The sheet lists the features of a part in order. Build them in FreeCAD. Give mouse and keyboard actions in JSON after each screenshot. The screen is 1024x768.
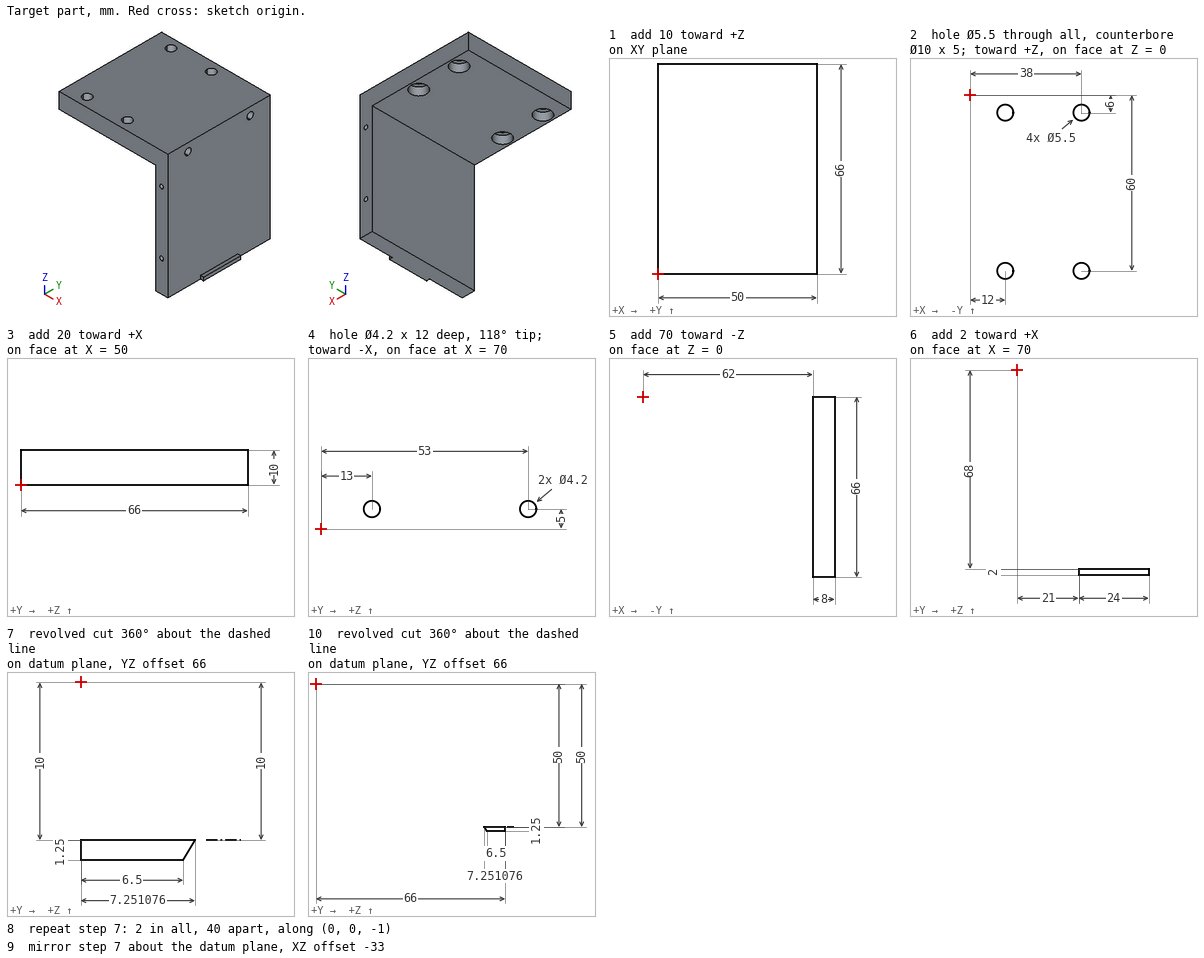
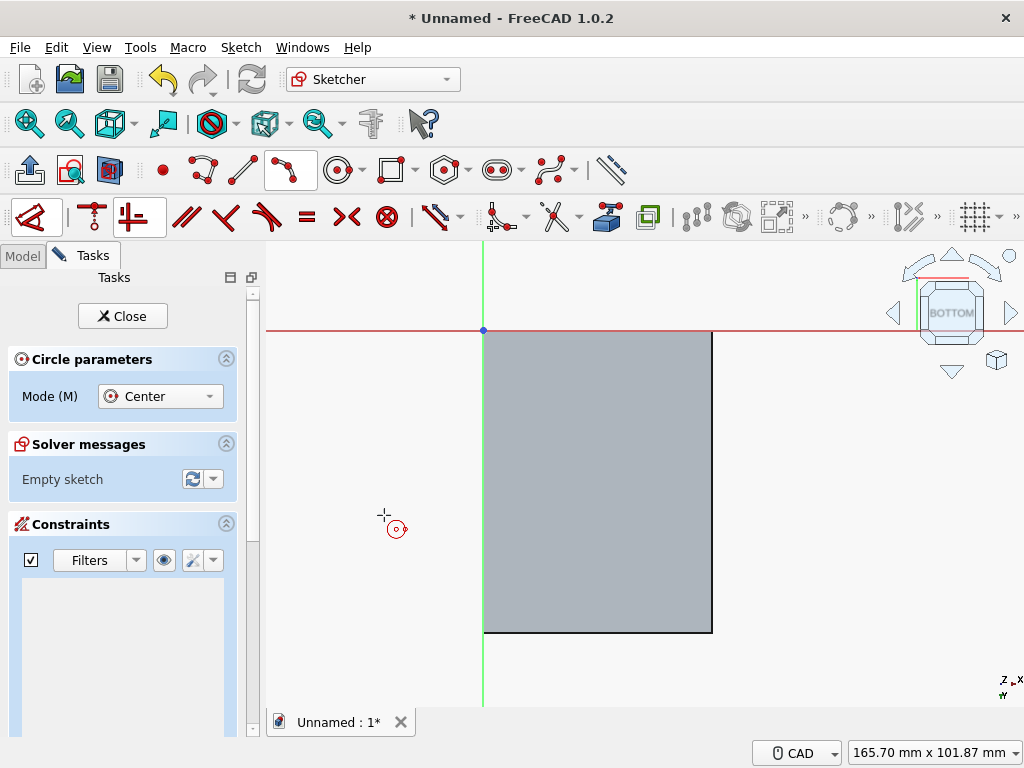
{"action": "scroll", "coordinate": [657, 358], "scroll_direction": "up", "scroll_amount": 3}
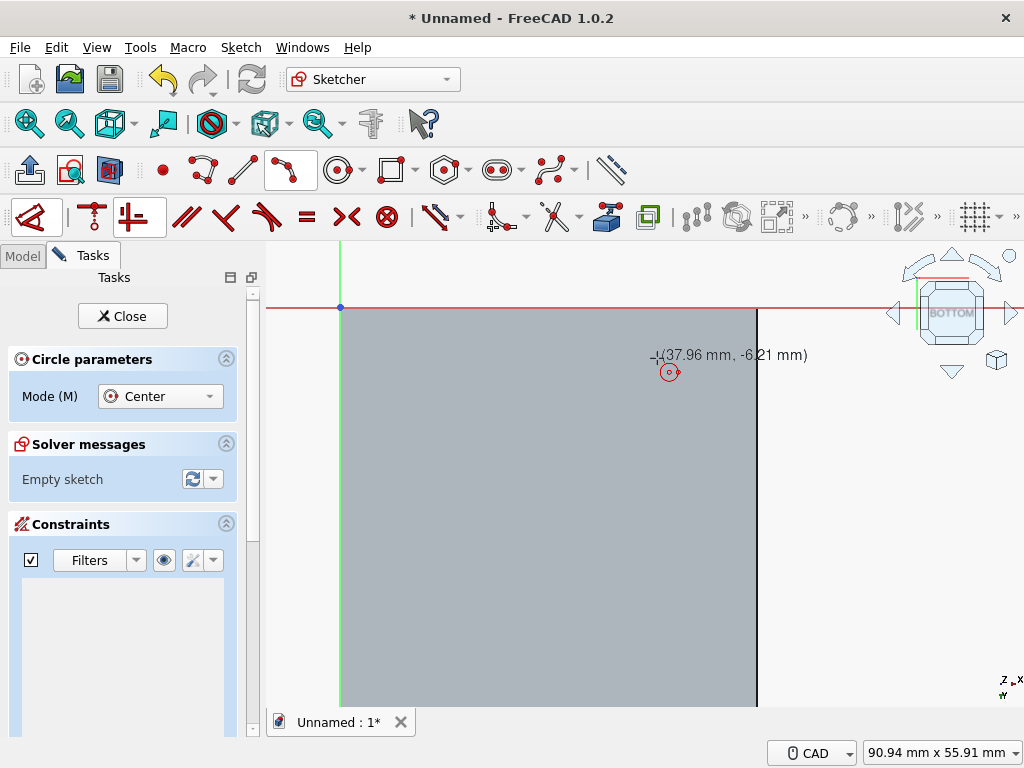
{"action": "left_click", "coordinate": [657, 358]}
{"action": "left_click", "coordinate": [673, 342]}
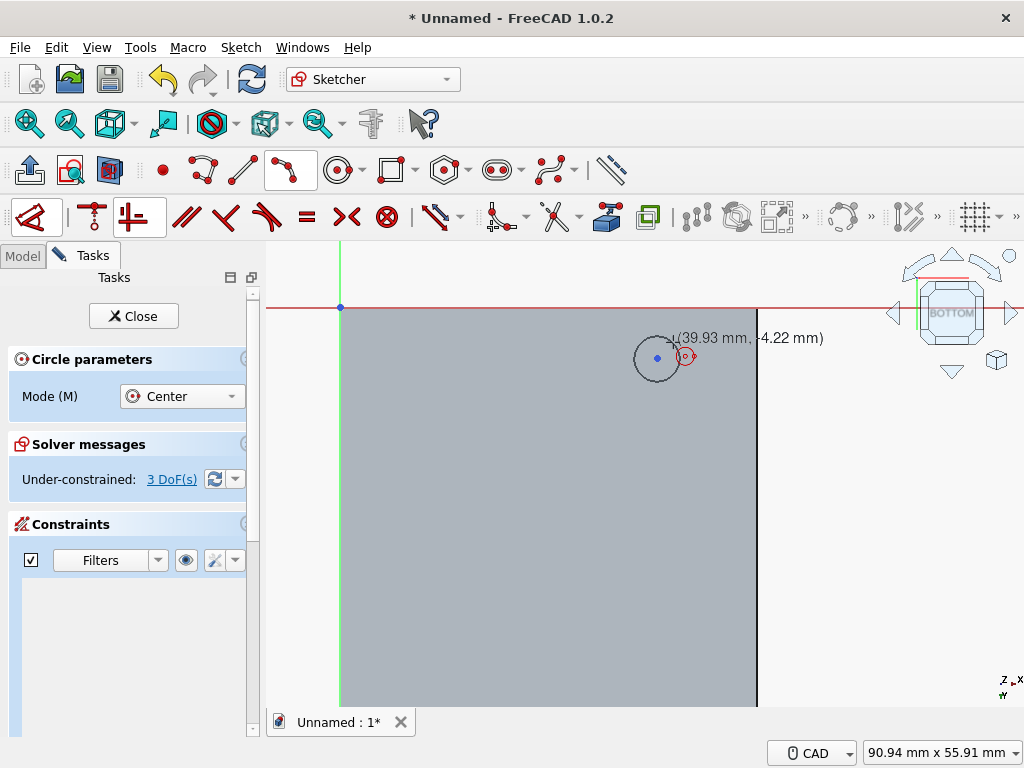
{"action": "scroll", "coordinate": [657, 358], "scroll_direction": "down", "scroll_amount": 3}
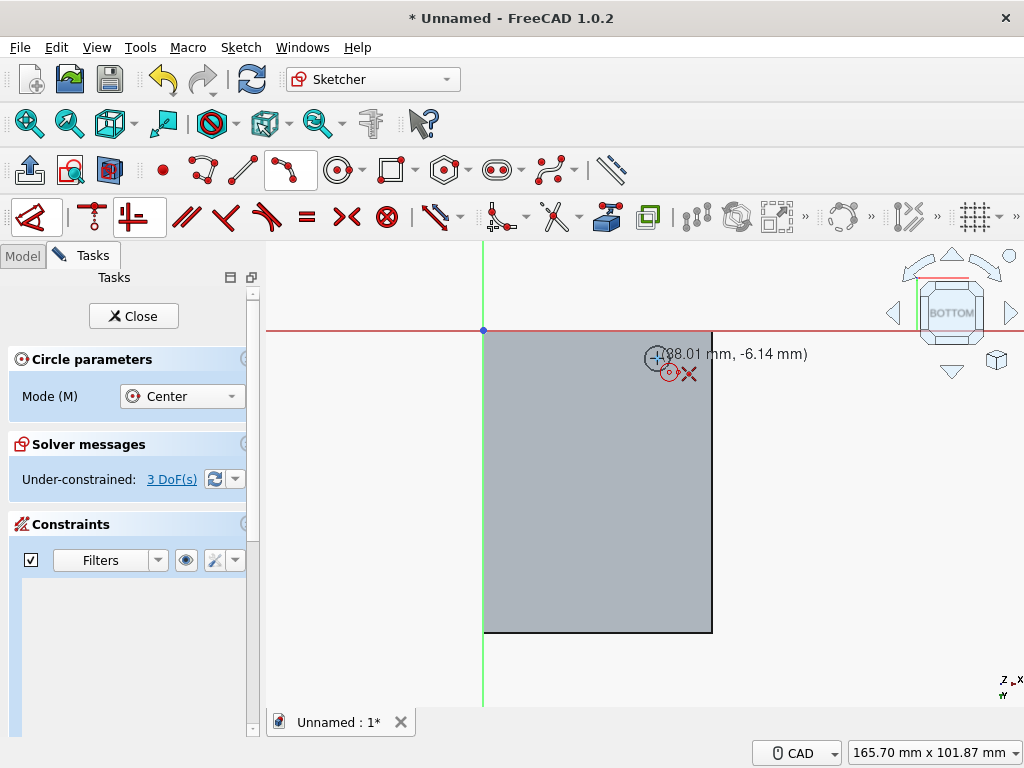
{"action": "scroll", "coordinate": [657, 605], "scroll_direction": "up", "scroll_amount": 3}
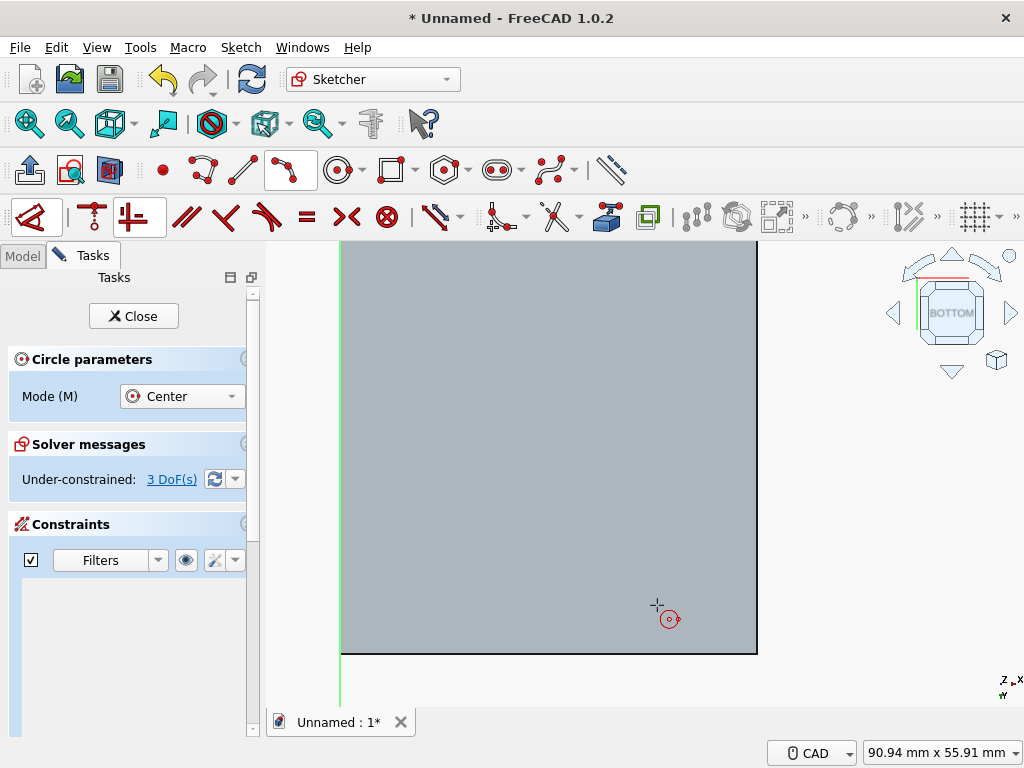
{"action": "left_click", "coordinate": [657, 604]}
{"action": "left_click", "coordinate": [673, 588]}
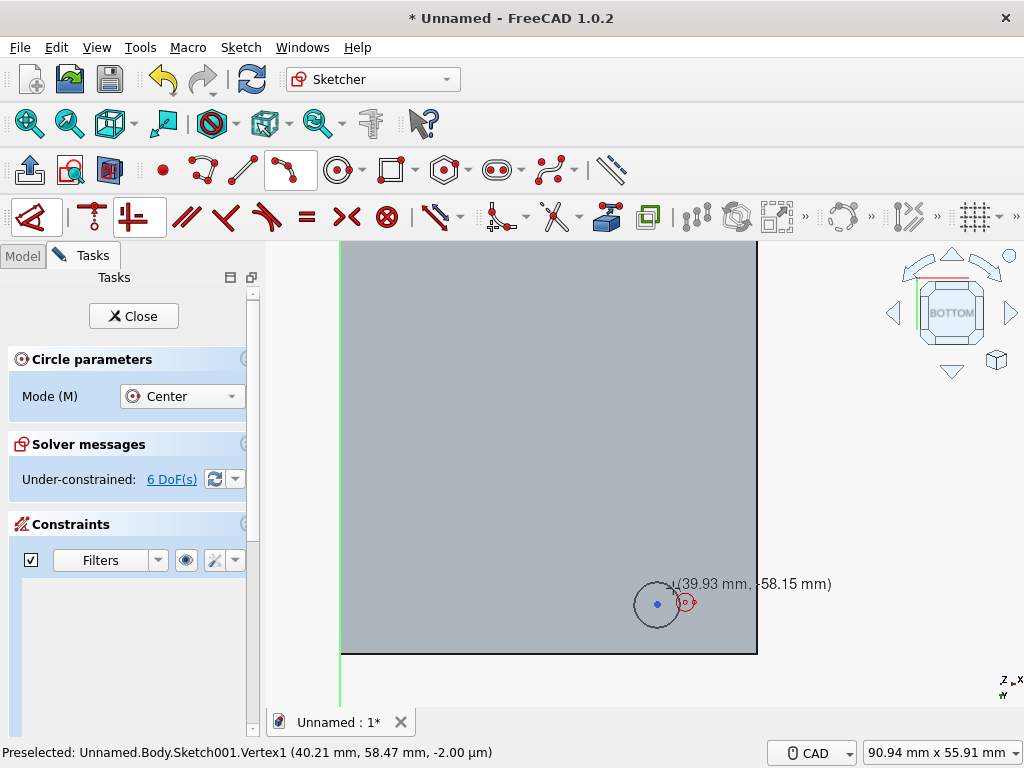
{"action": "left_click", "coordinate": [440, 604]}
{"action": "left_click", "coordinate": [456, 588]}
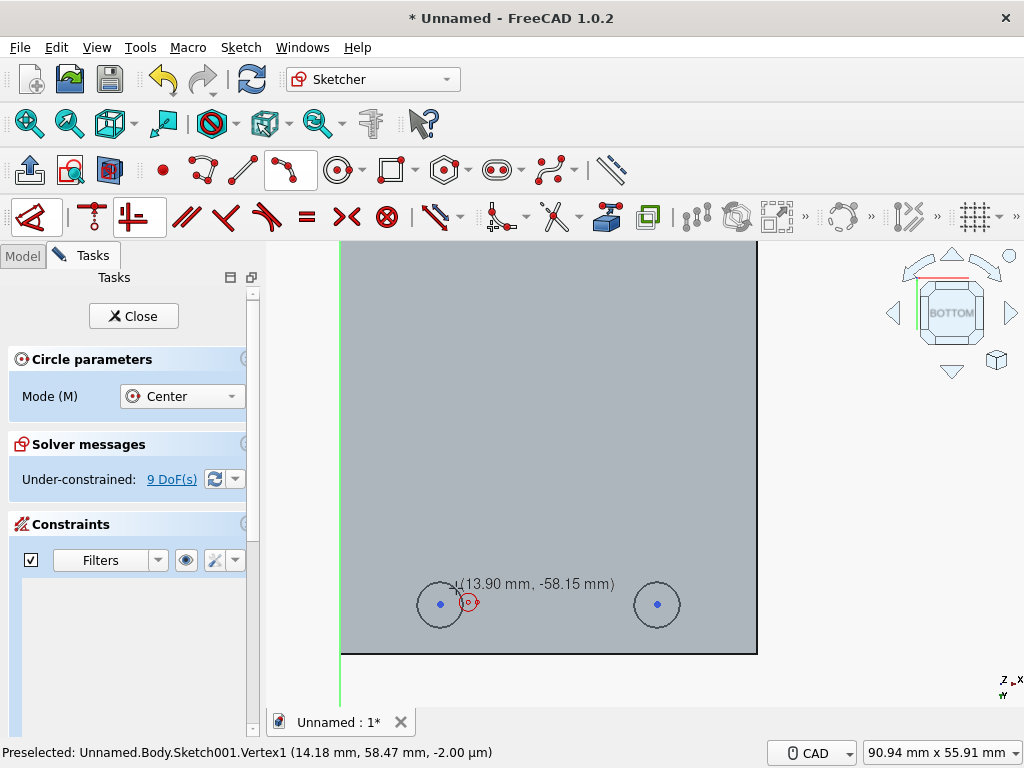
{"action": "scroll", "coordinate": [657, 606], "scroll_direction": "down", "scroll_amount": 3}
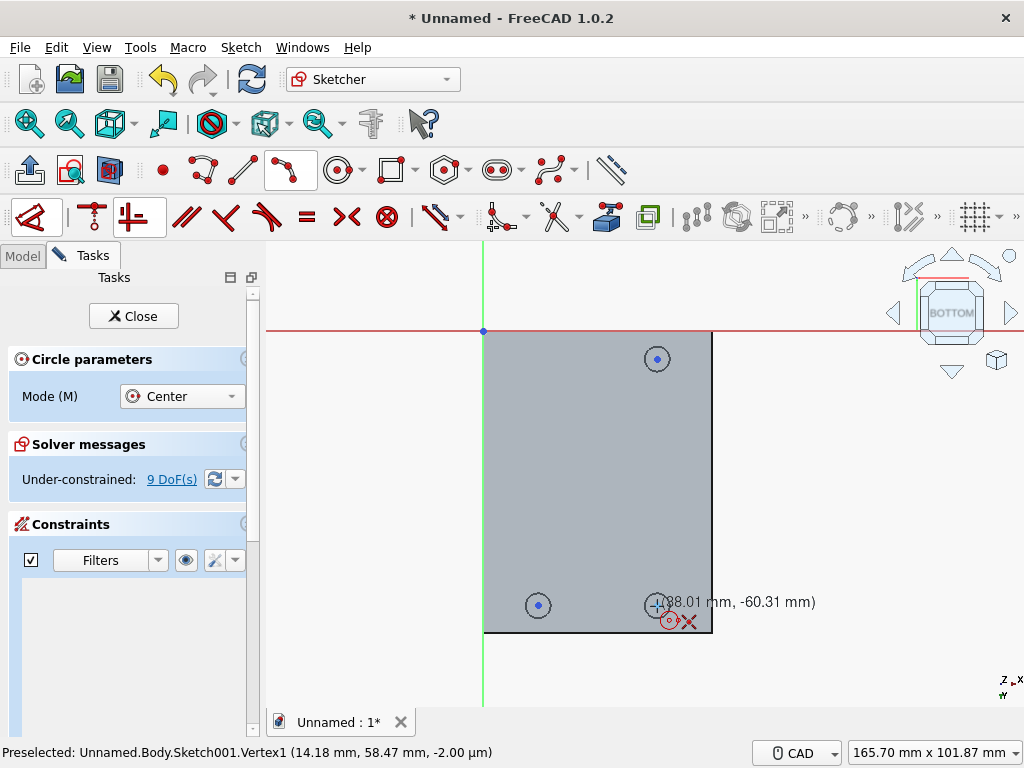
{"action": "scroll", "coordinate": [538, 358], "scroll_direction": "up", "scroll_amount": 3}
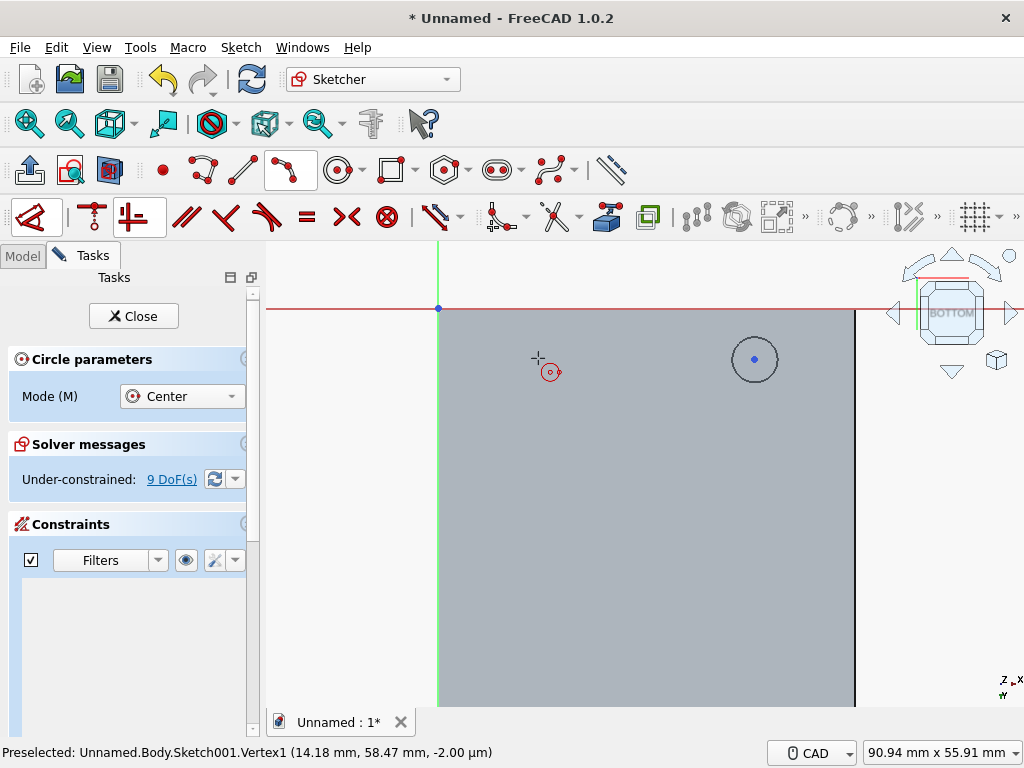
{"action": "left_click", "coordinate": [538, 359]}
{"action": "left_click", "coordinate": [554, 342]}
{"action": "key", "text": "Escape"}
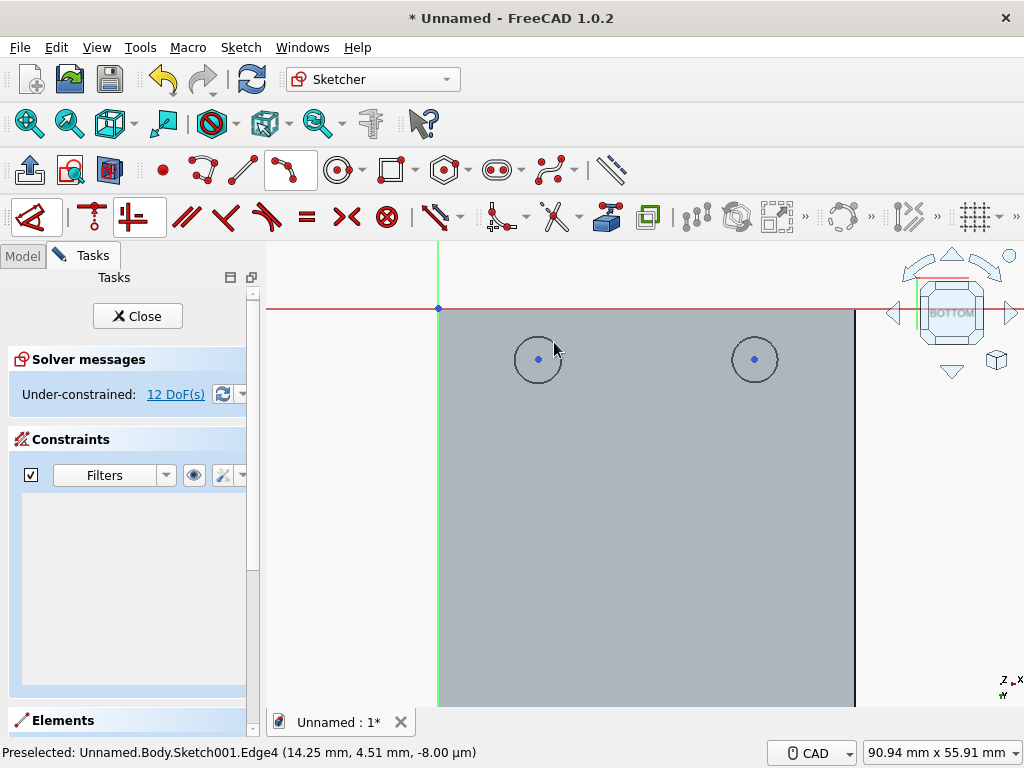
{"action": "left_click", "coordinate": [771, 344]}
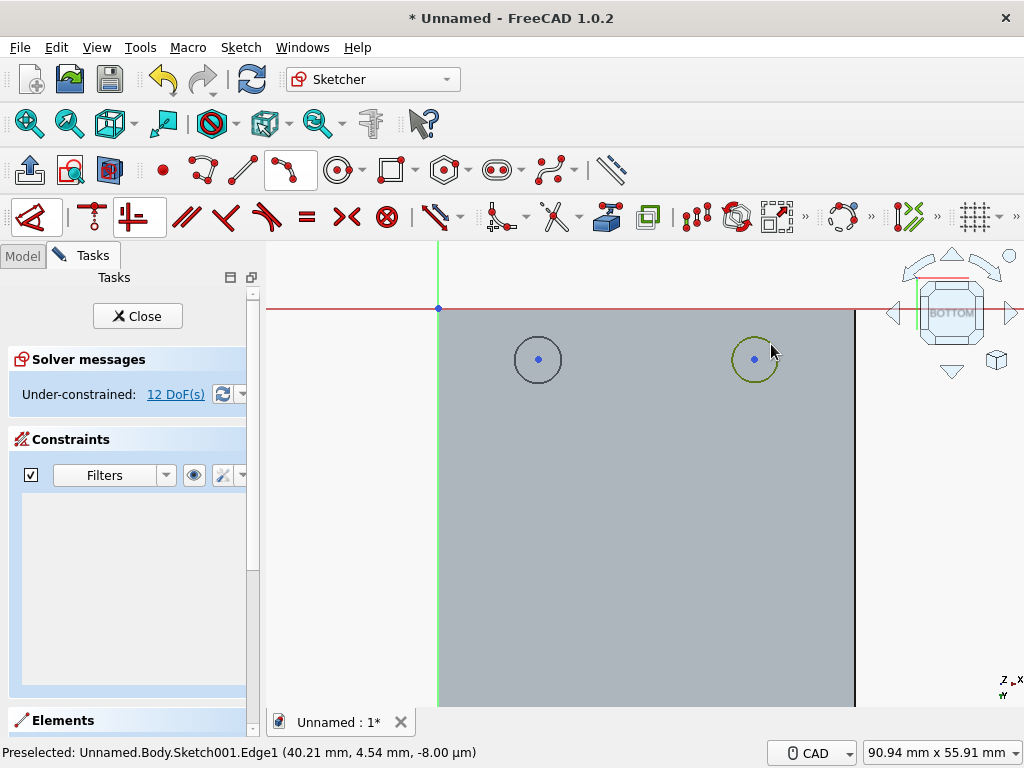
{"action": "scroll", "coordinate": [538, 357], "scroll_direction": "down", "scroll_amount": 3}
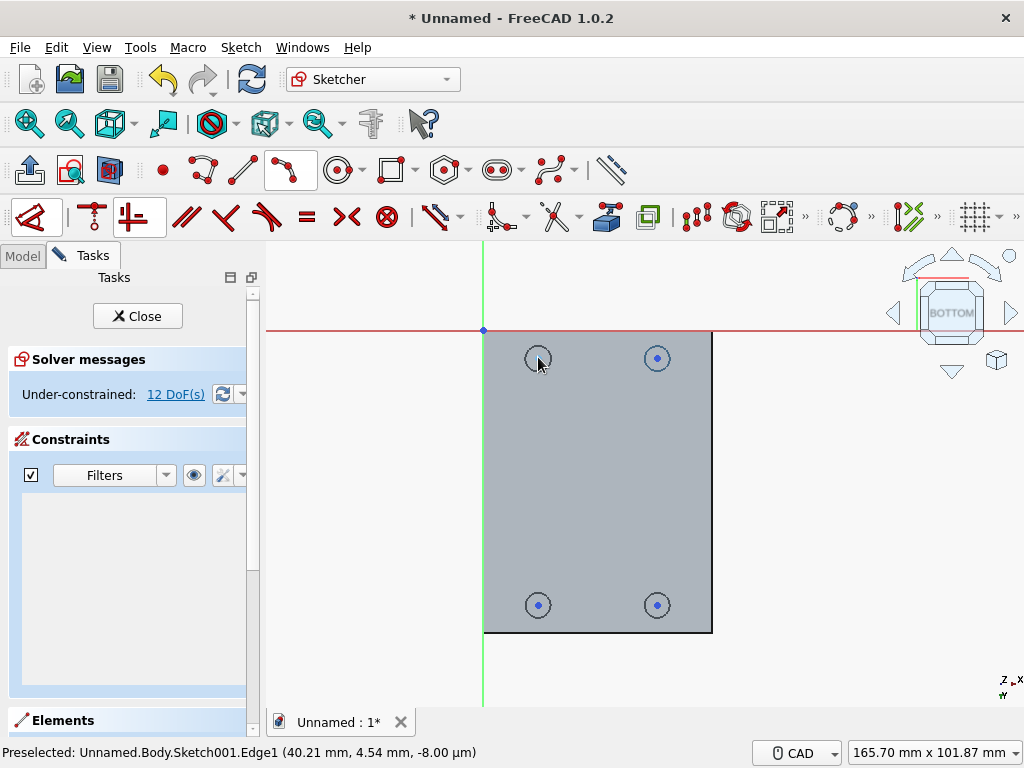
{"action": "left_click", "coordinate": [666, 597]}